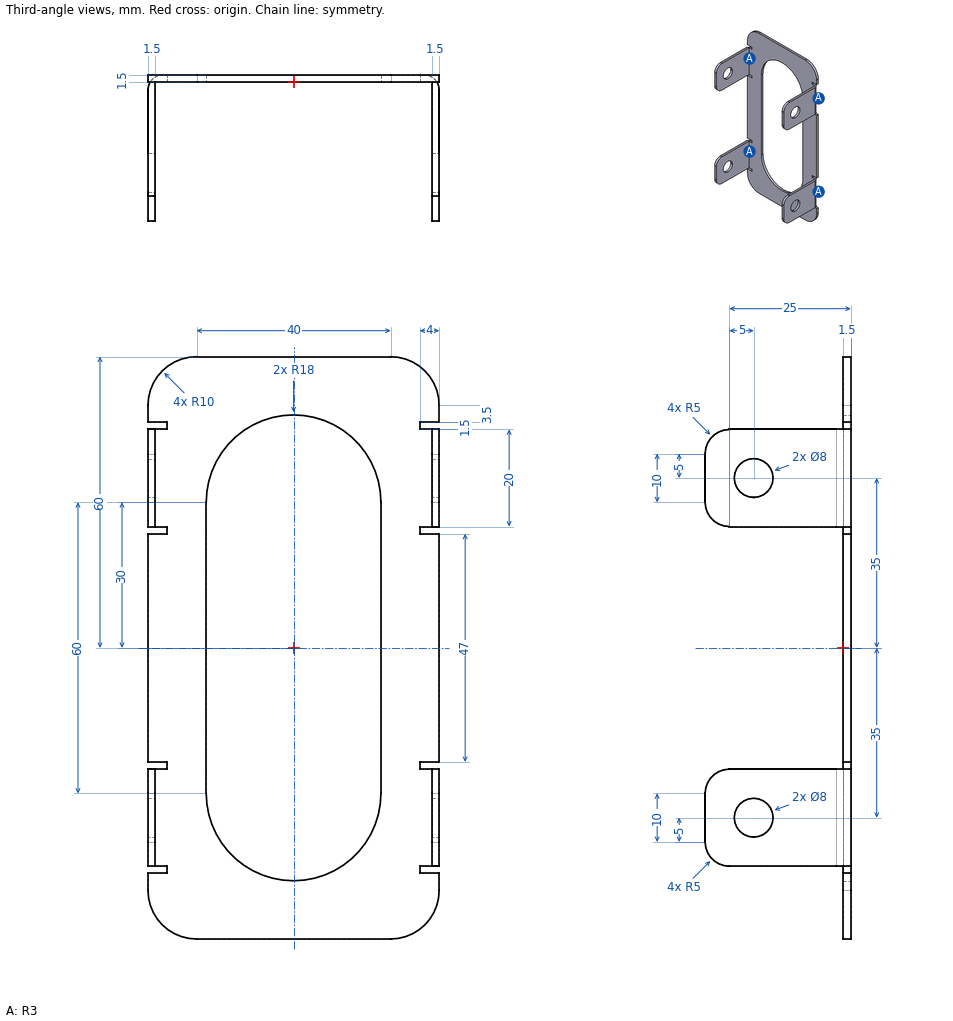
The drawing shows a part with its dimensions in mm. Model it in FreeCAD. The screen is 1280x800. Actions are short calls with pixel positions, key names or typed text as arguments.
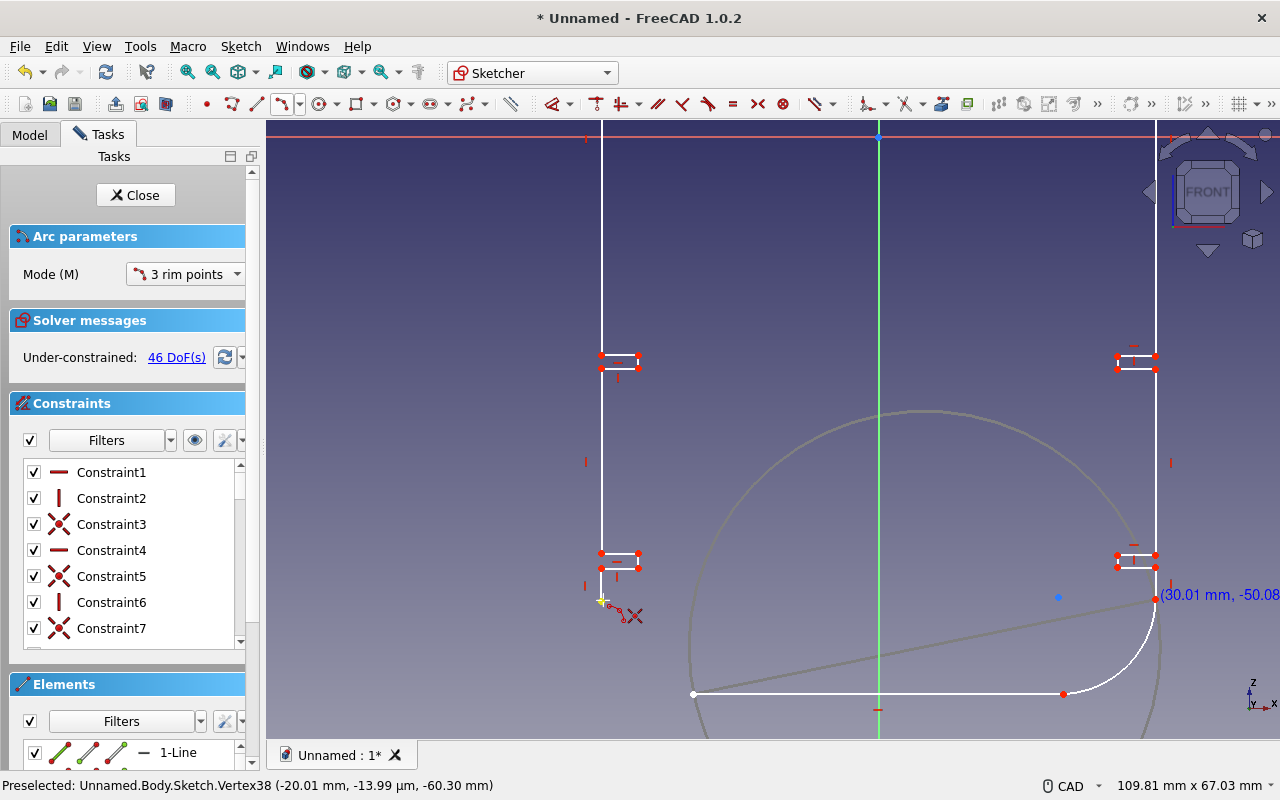
click(601, 602)
click(629, 664)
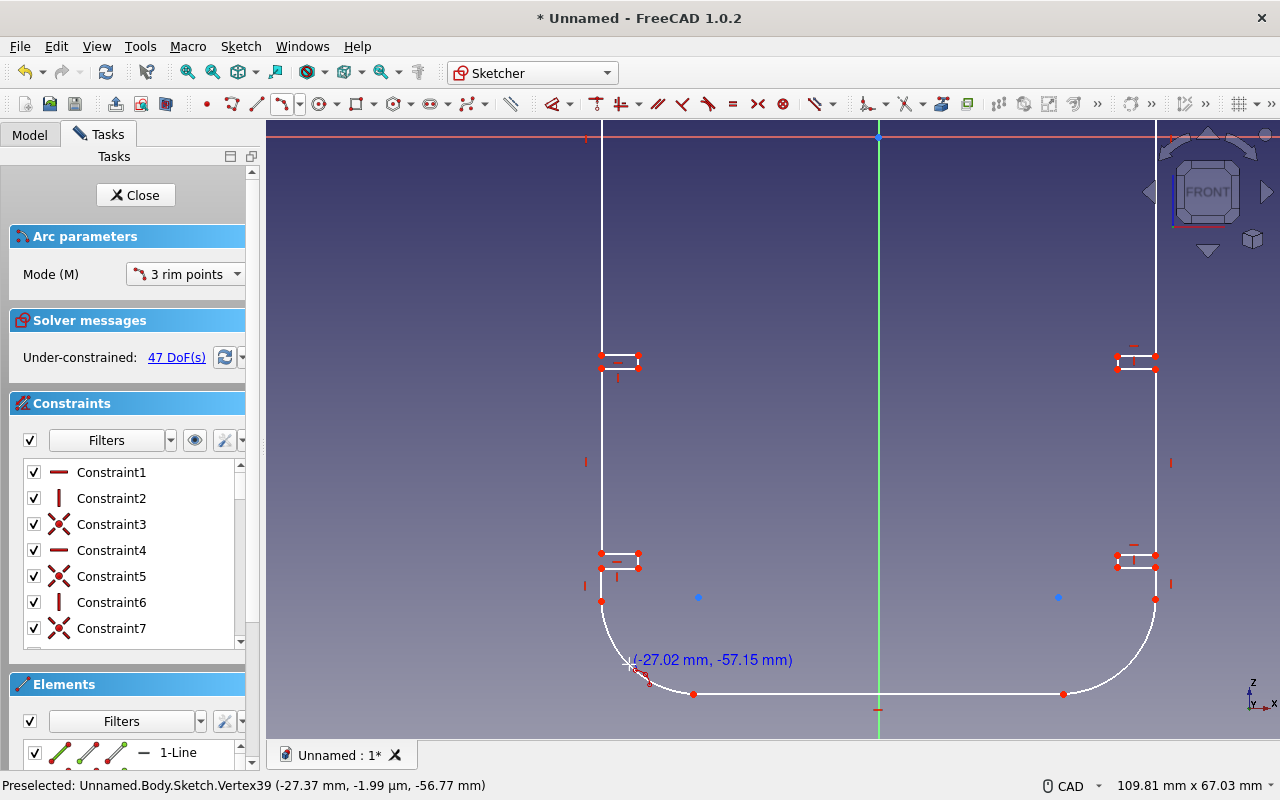
scroll(603, 600, down, 5)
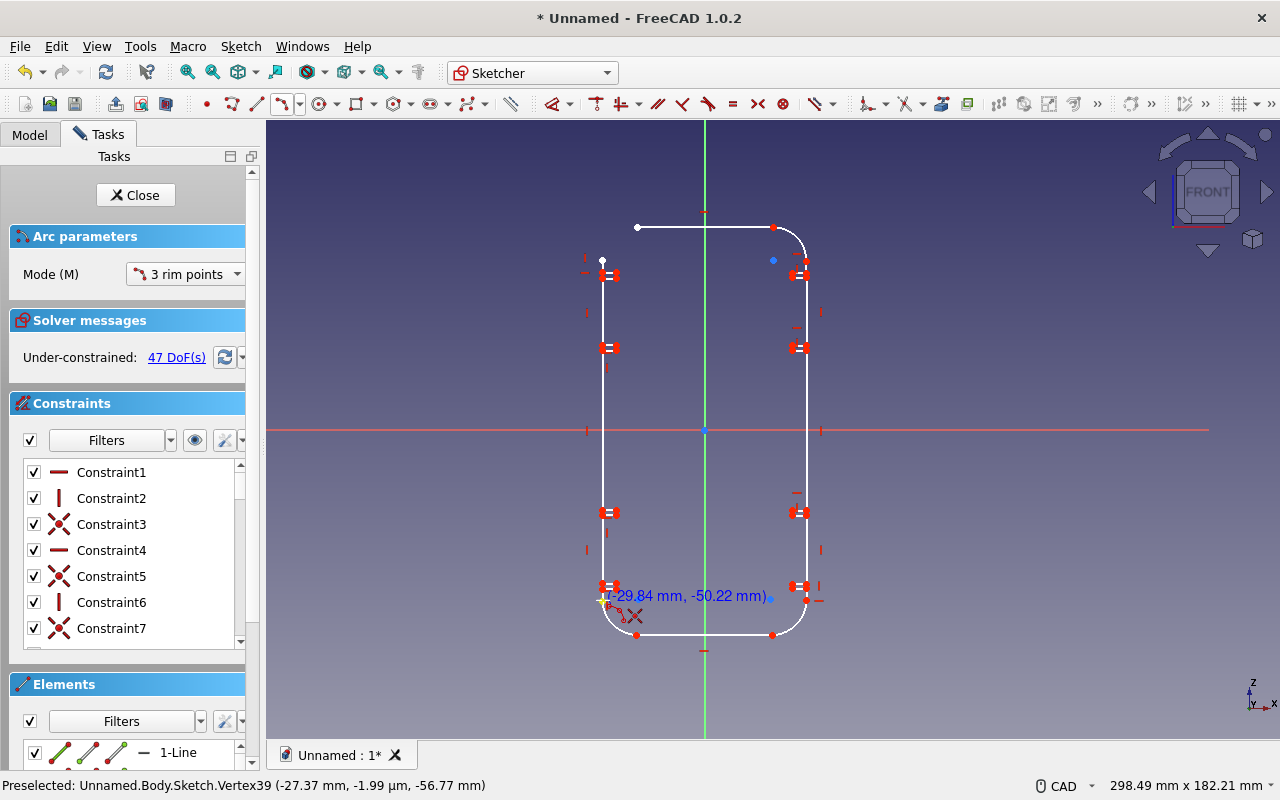
scroll(603, 260, up, 5)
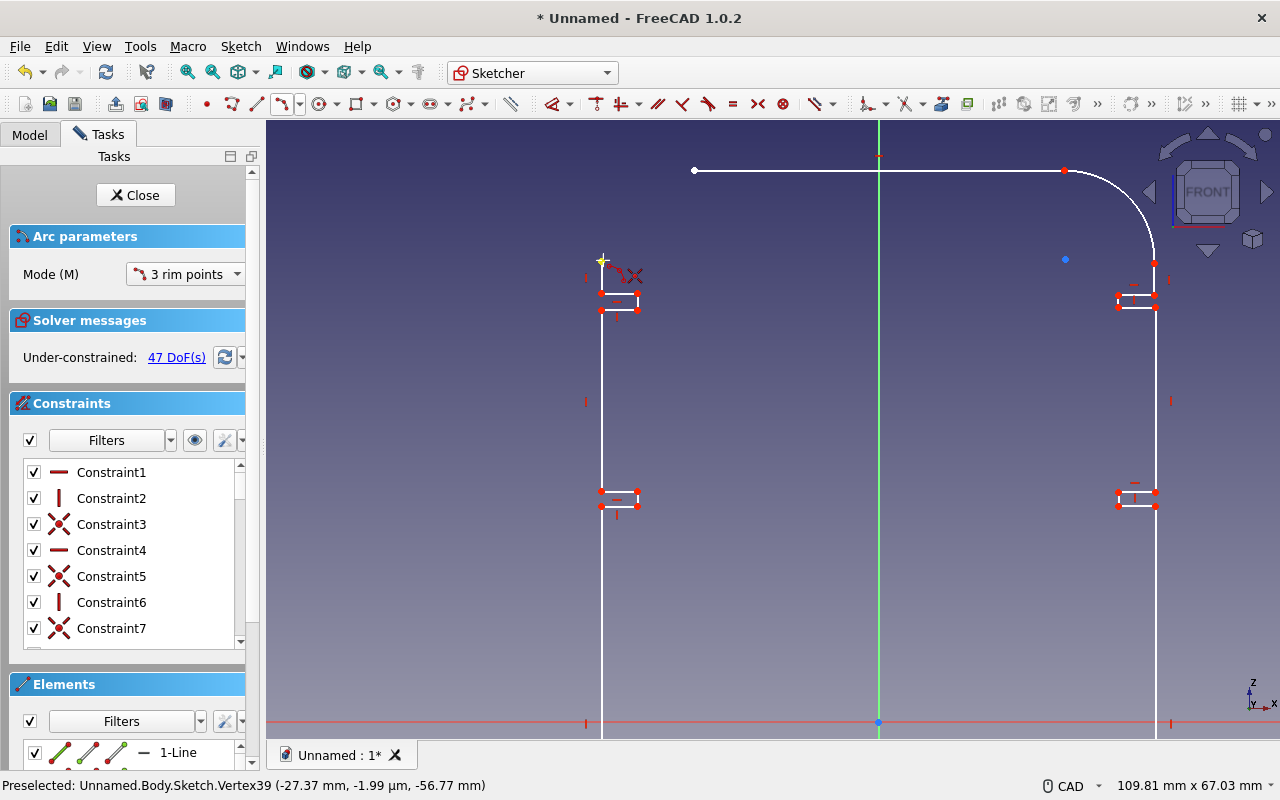
click(602, 262)
click(695, 171)
click(629, 195)
key(Escape)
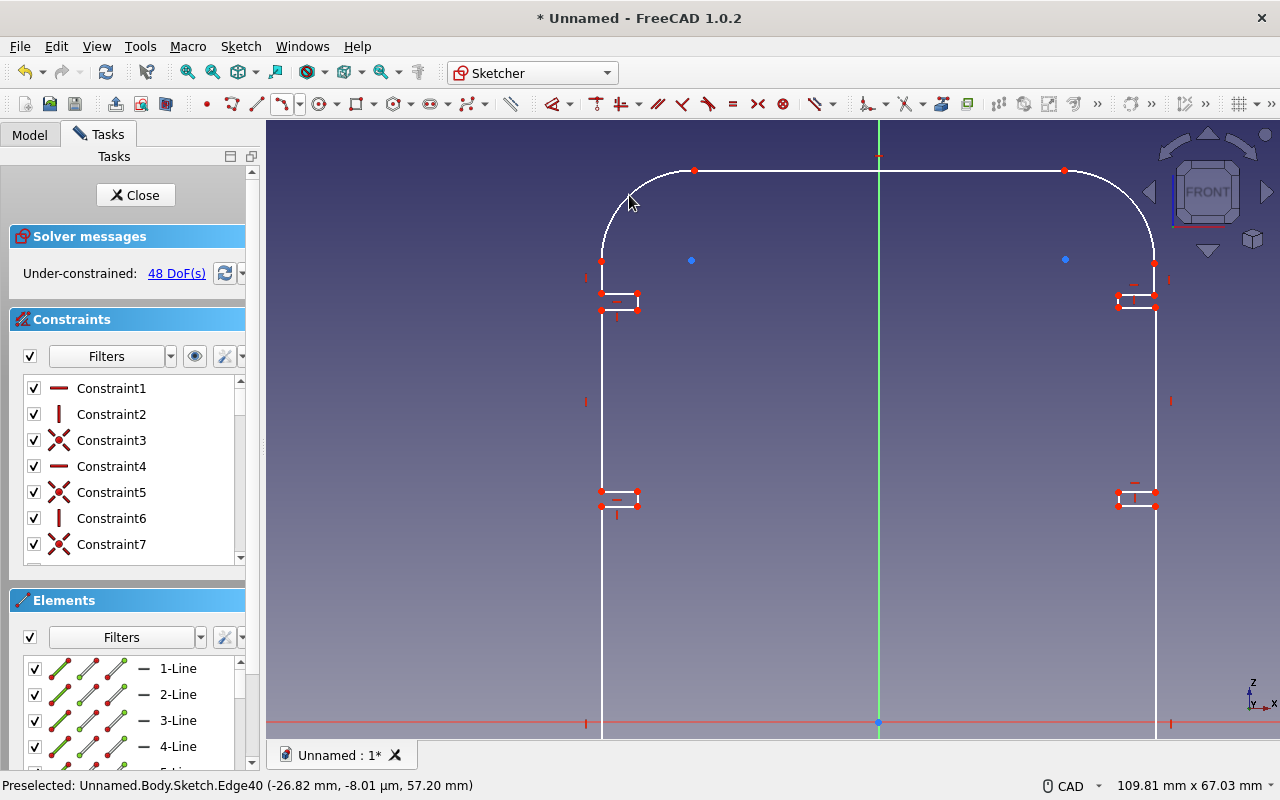
click(806, 171)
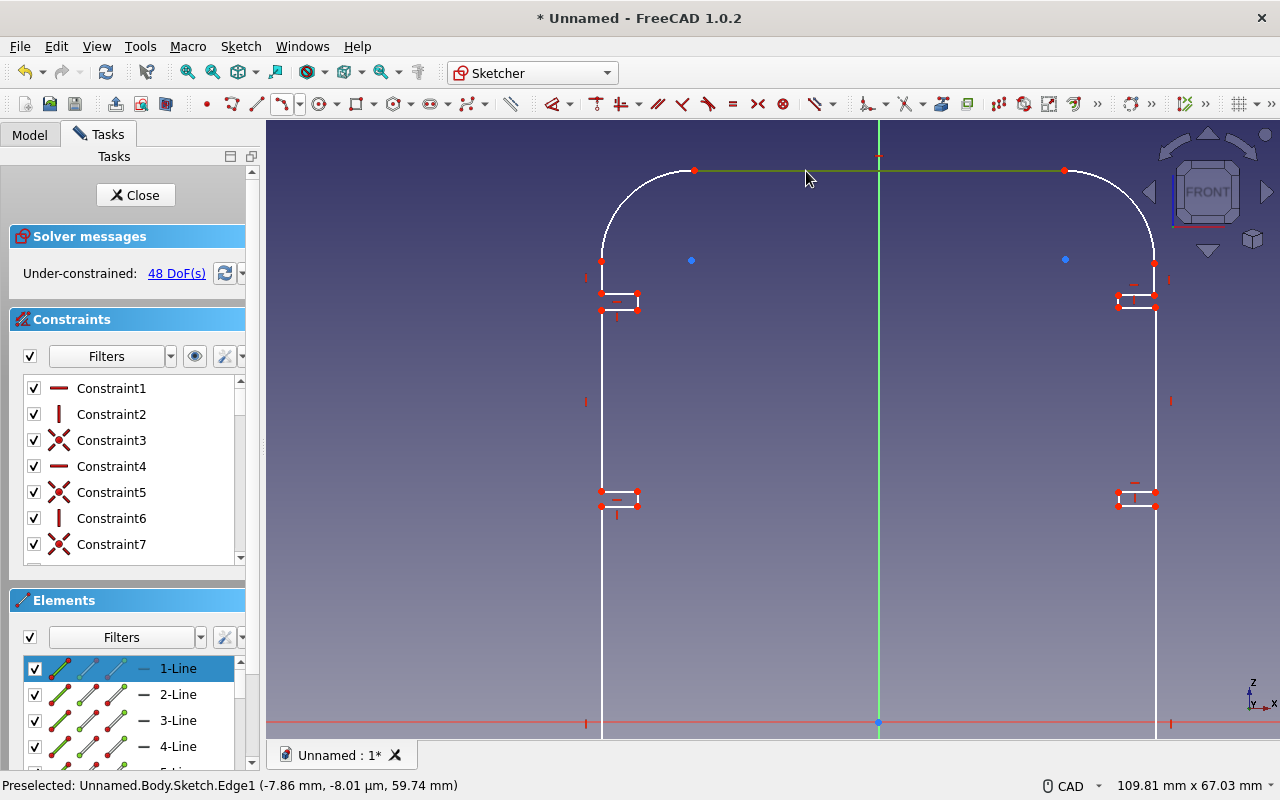
click(1106, 181)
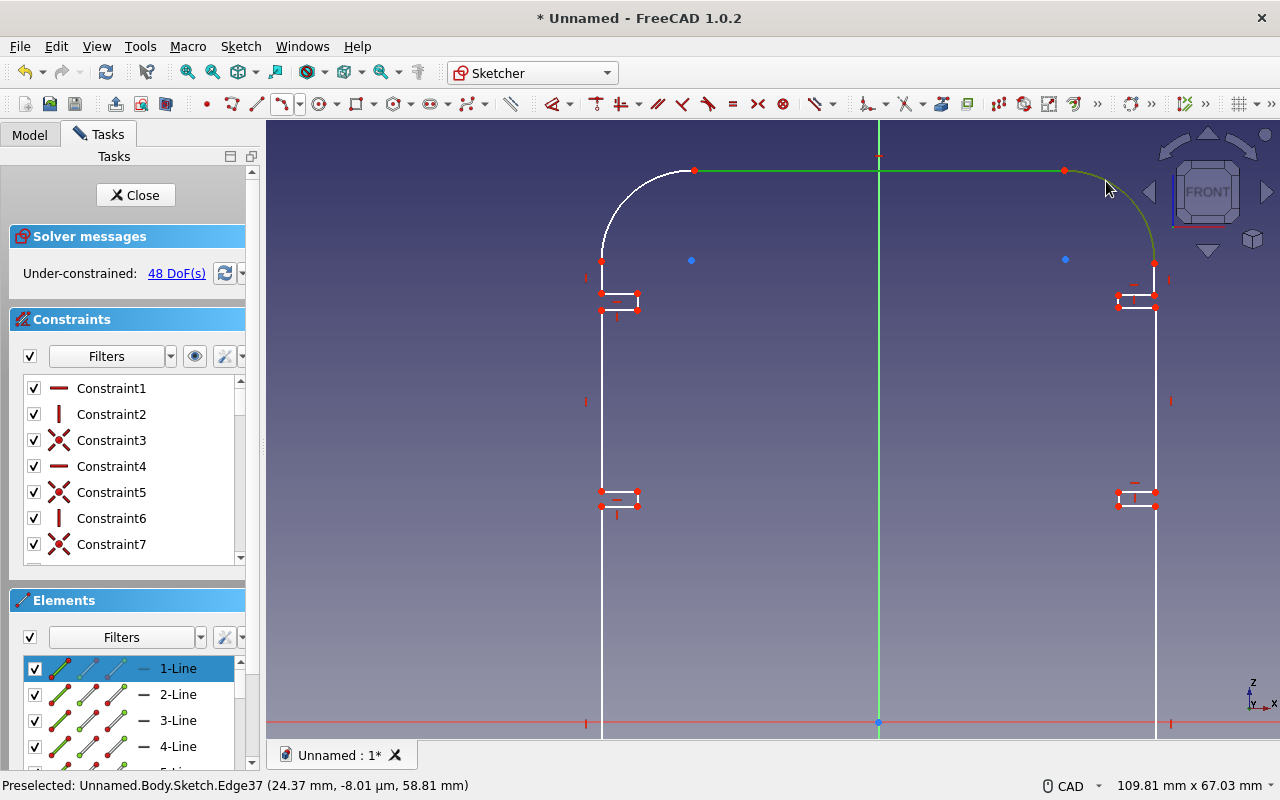
click(708, 104)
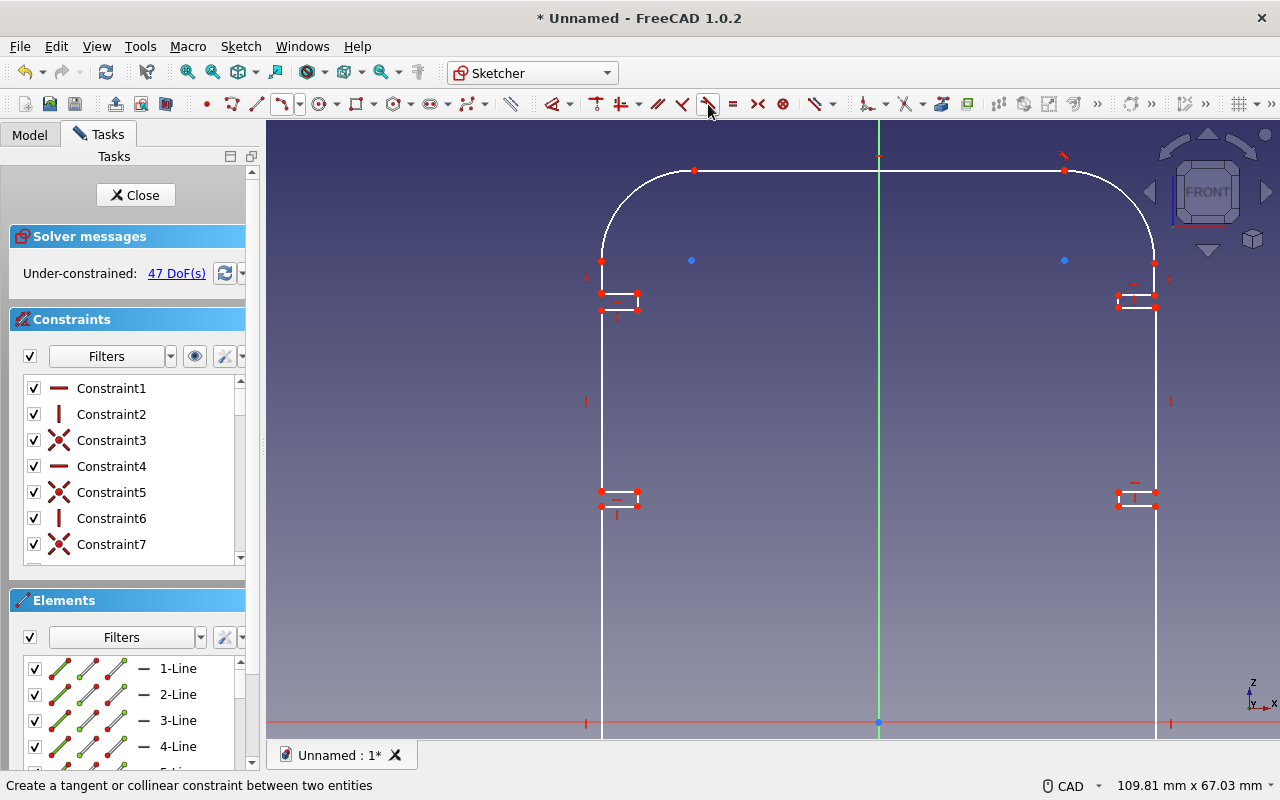
click(806, 171)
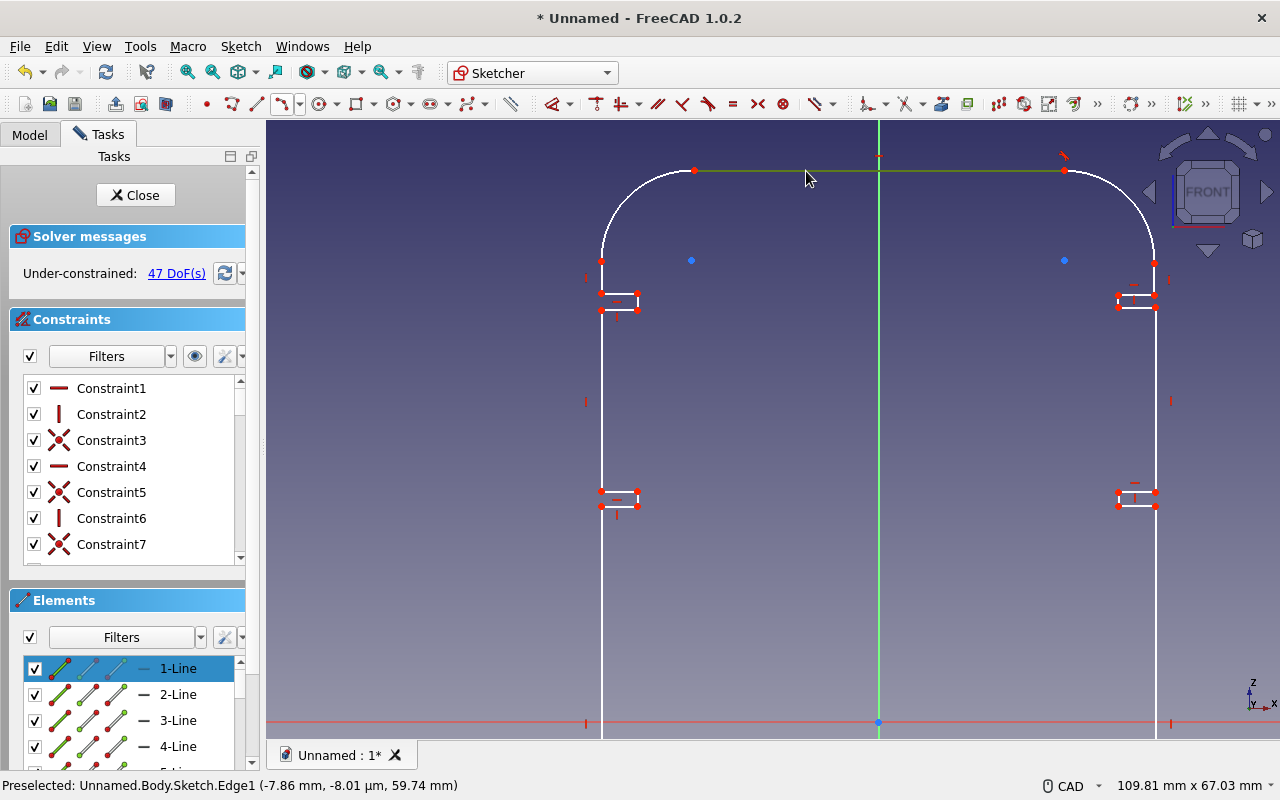
click(653, 180)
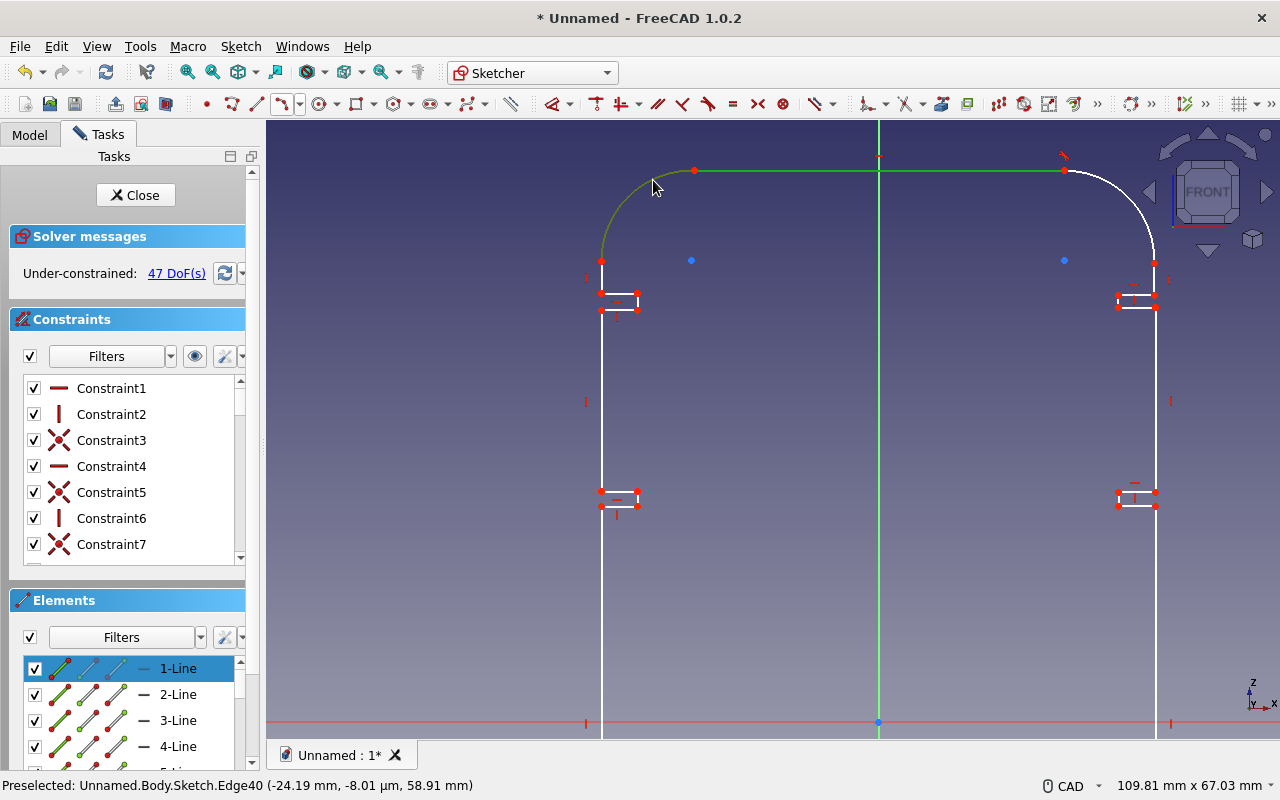
click(708, 104)